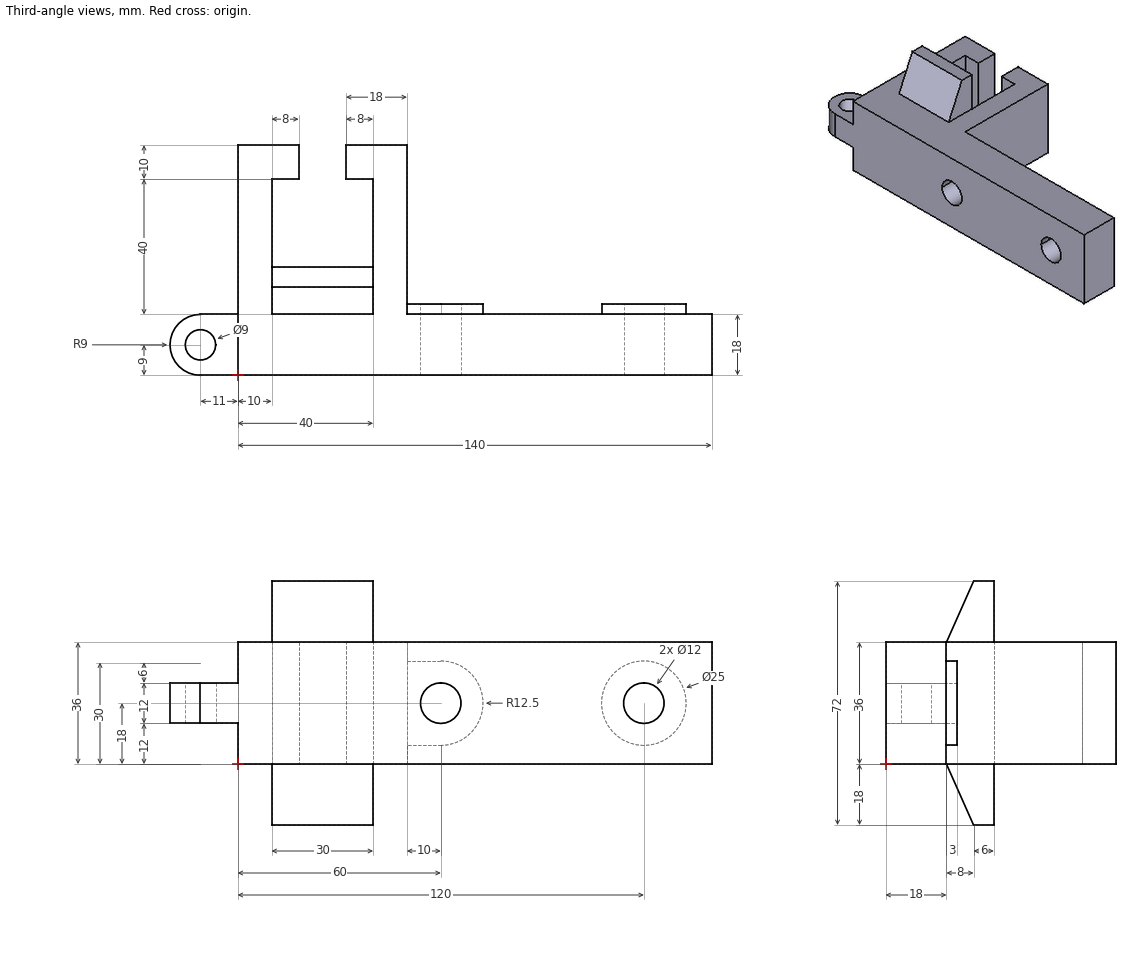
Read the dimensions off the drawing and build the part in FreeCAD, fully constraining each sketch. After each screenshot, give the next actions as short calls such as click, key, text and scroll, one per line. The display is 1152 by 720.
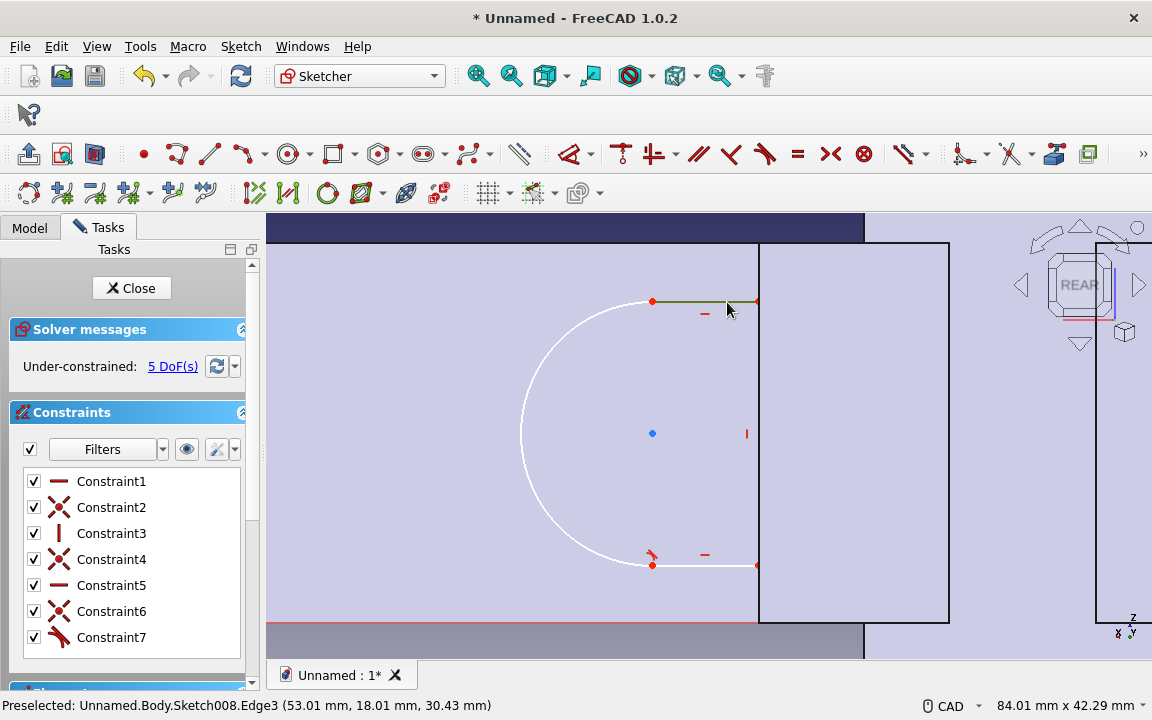
click(546, 356)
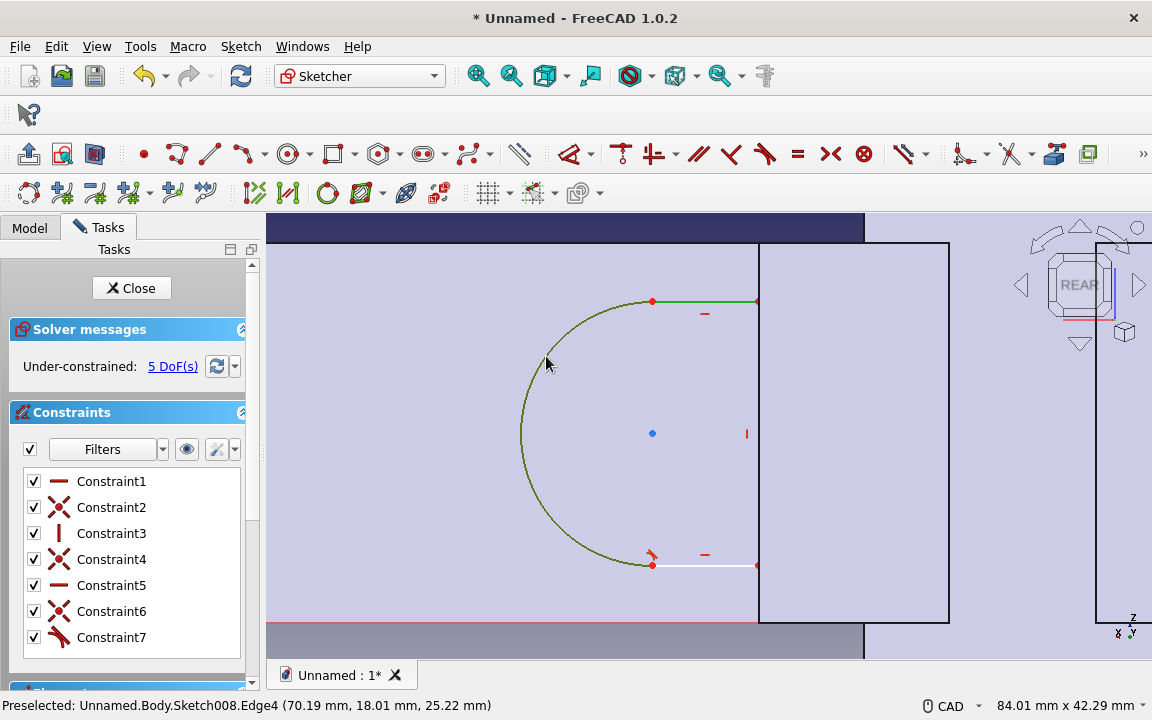
click(765, 154)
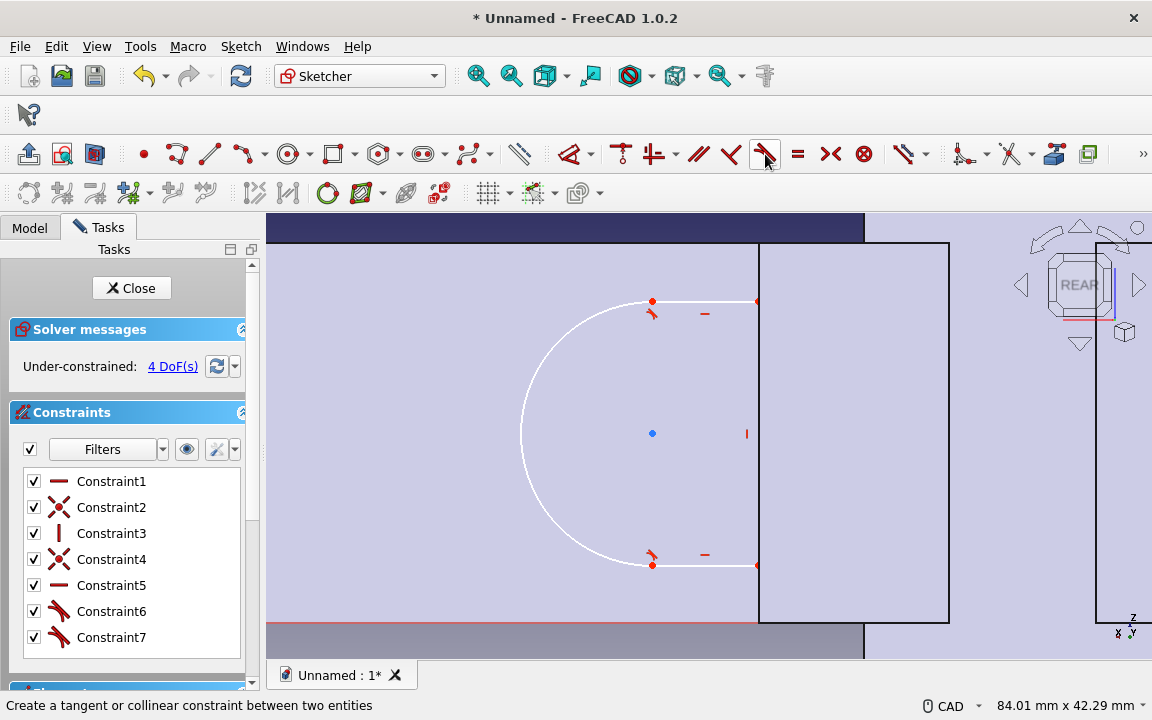
key(d)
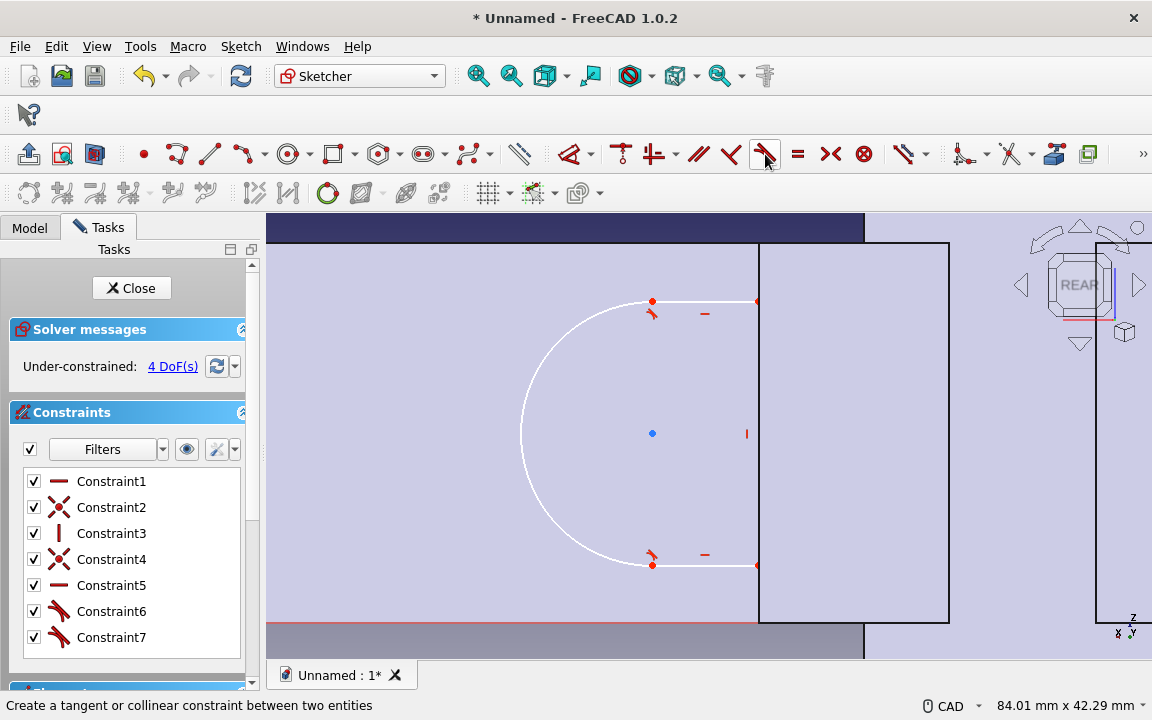
click(546, 356)
click(520, 337)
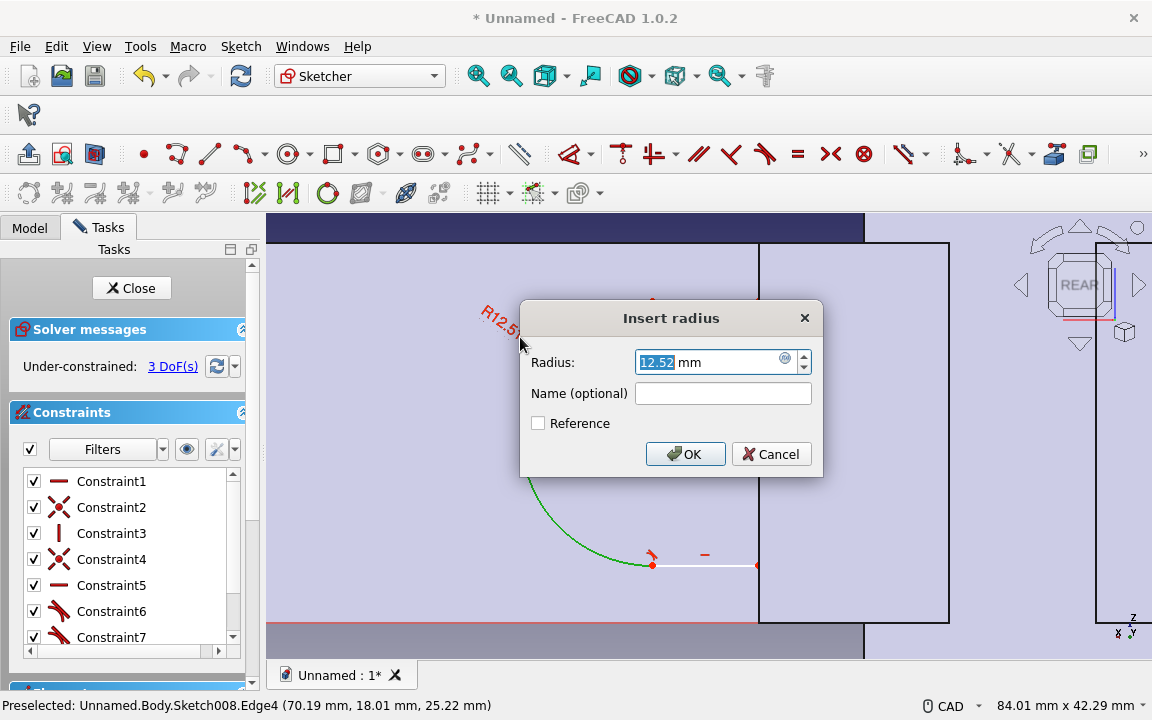
text(12.5)
key(Return)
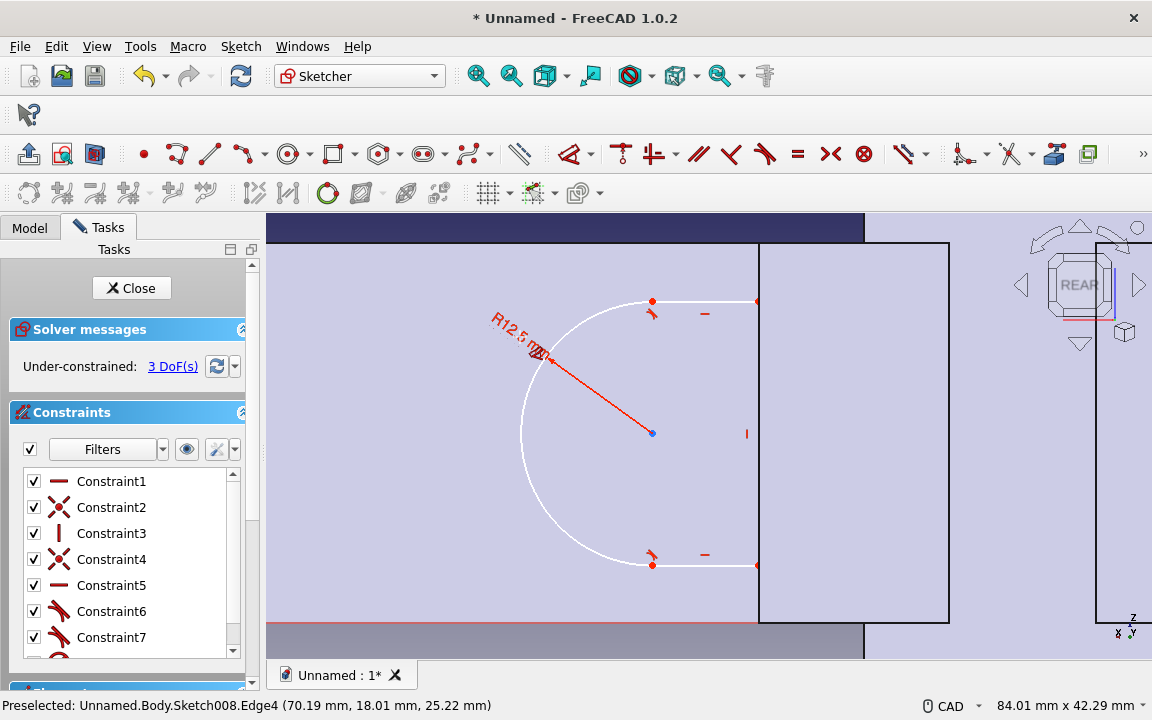
click(685, 566)
click(706, 600)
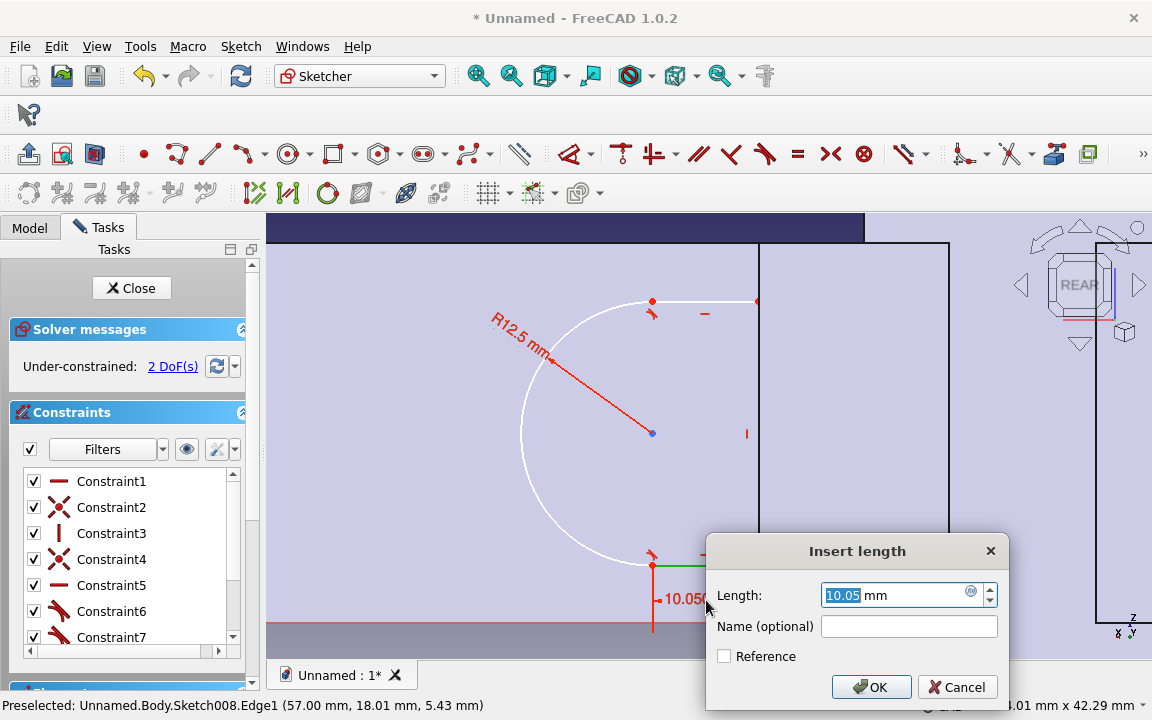
text(10)
key(Return)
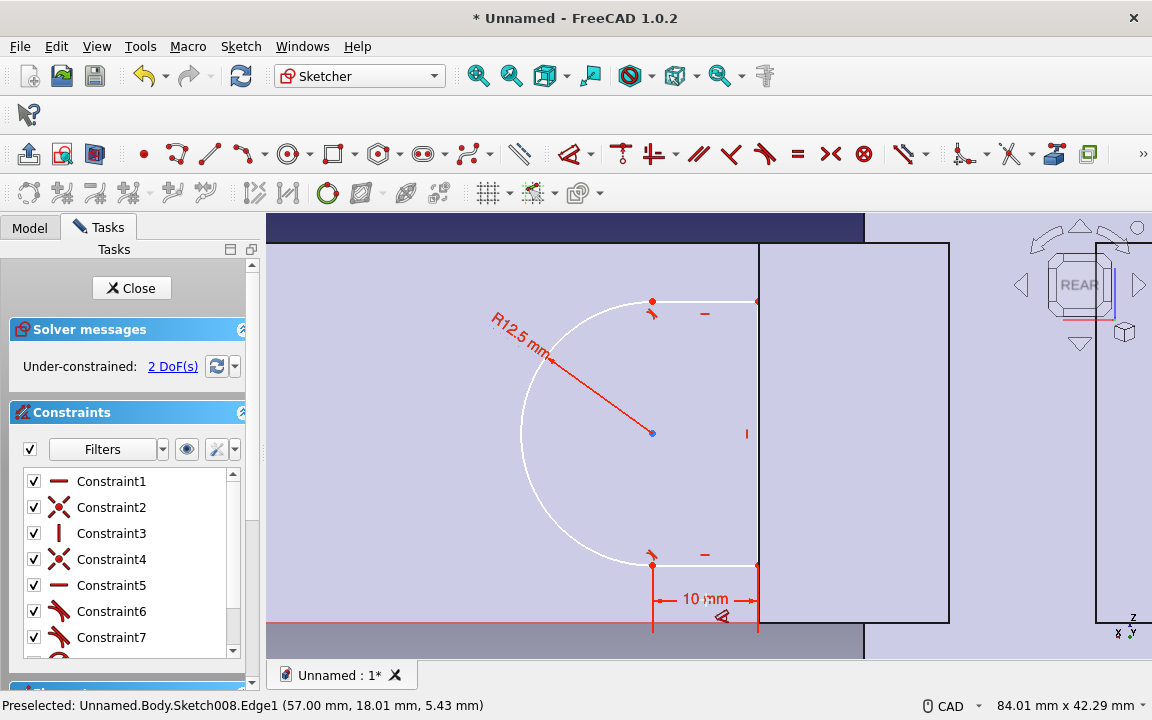
click(653, 566)
click(820, 532)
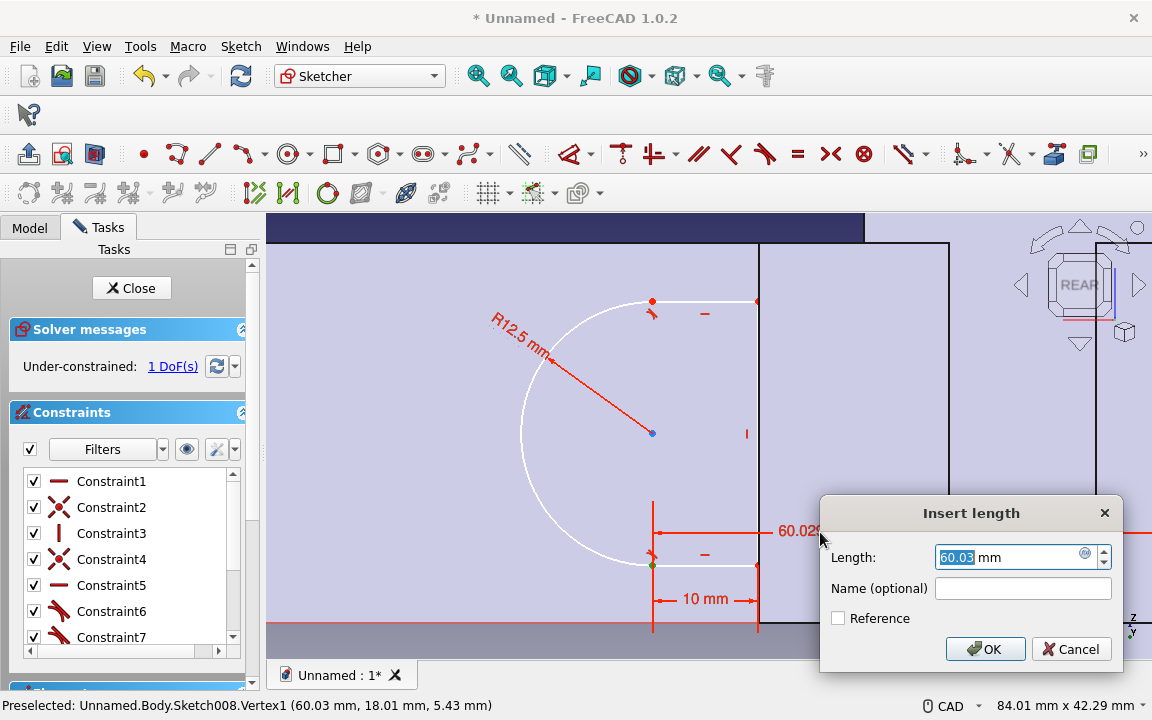
text(60)
key(Return)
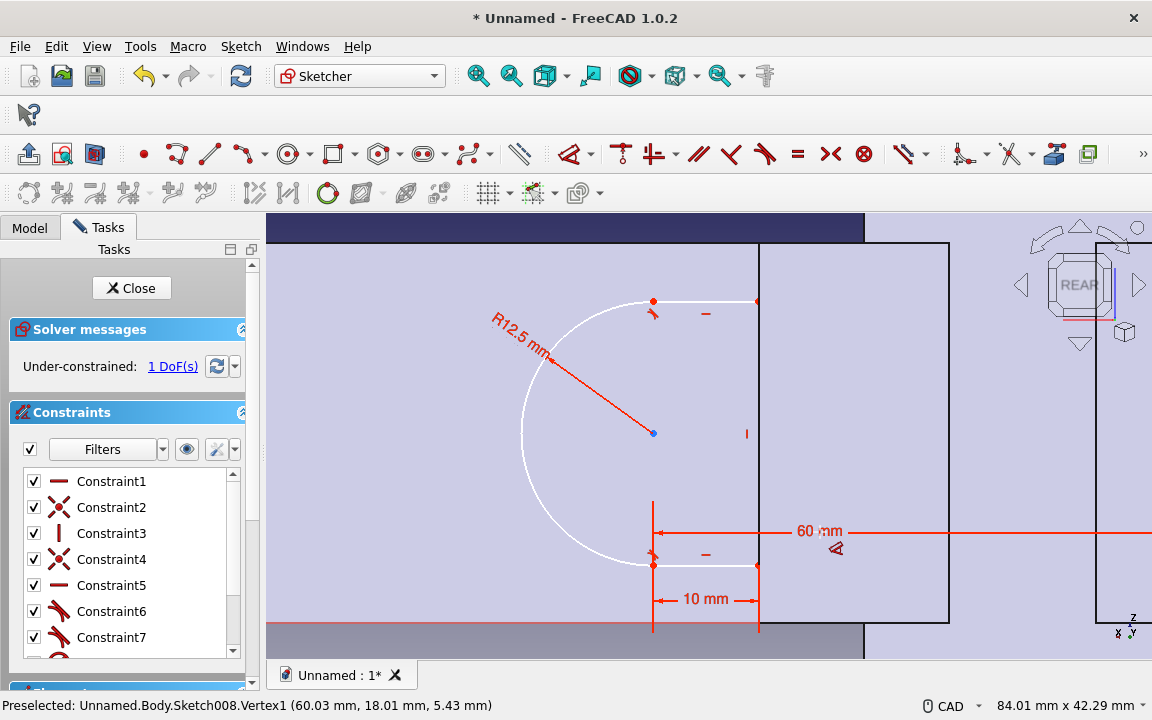
click(653, 434)
click(619, 528)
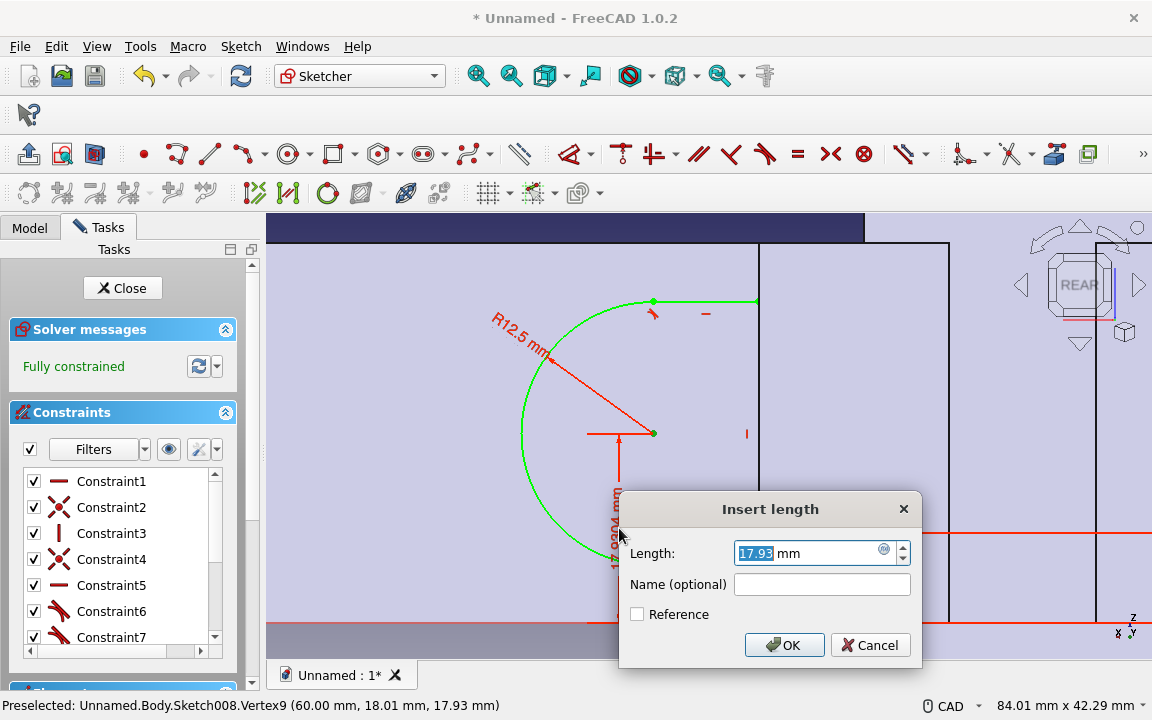
text(18)
key(Return)
key(Escape)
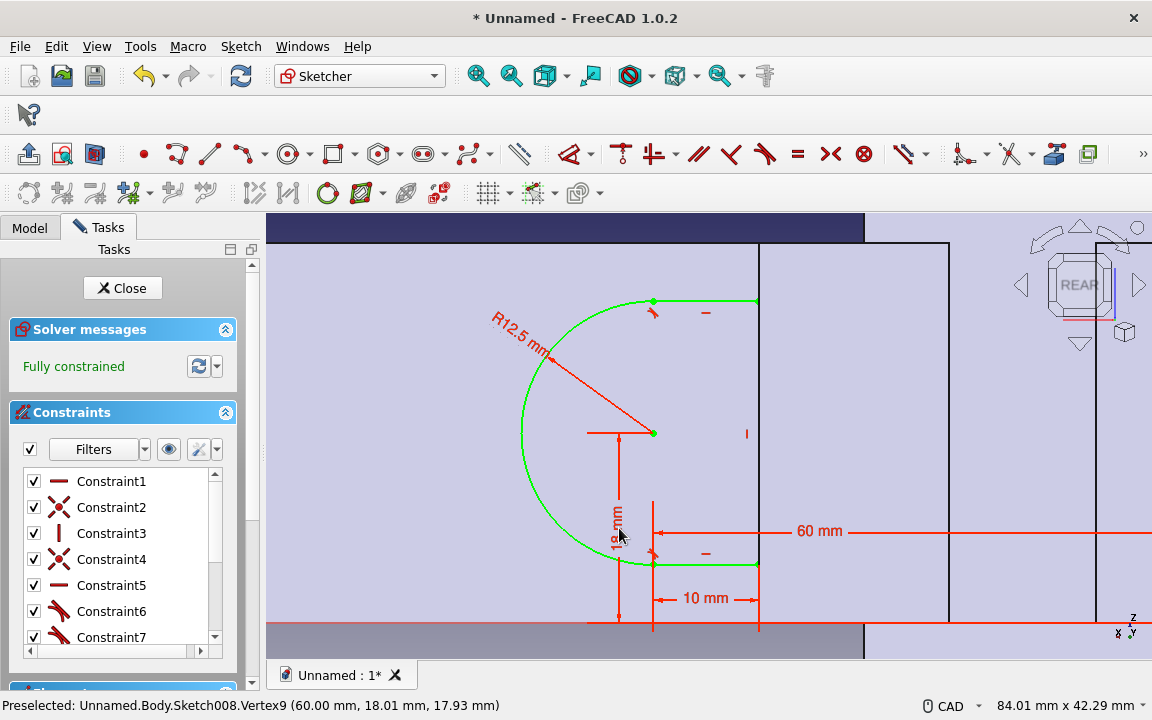
click(123, 288)